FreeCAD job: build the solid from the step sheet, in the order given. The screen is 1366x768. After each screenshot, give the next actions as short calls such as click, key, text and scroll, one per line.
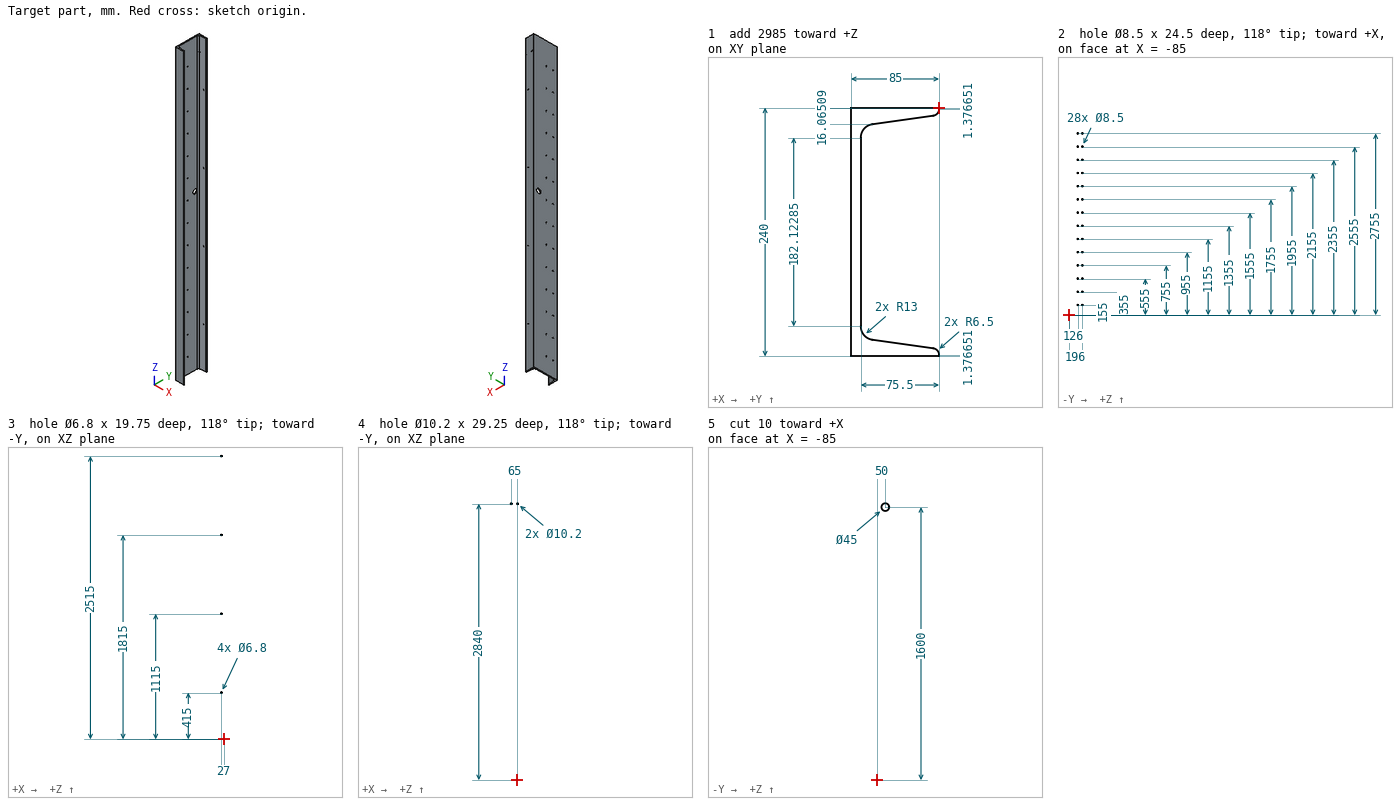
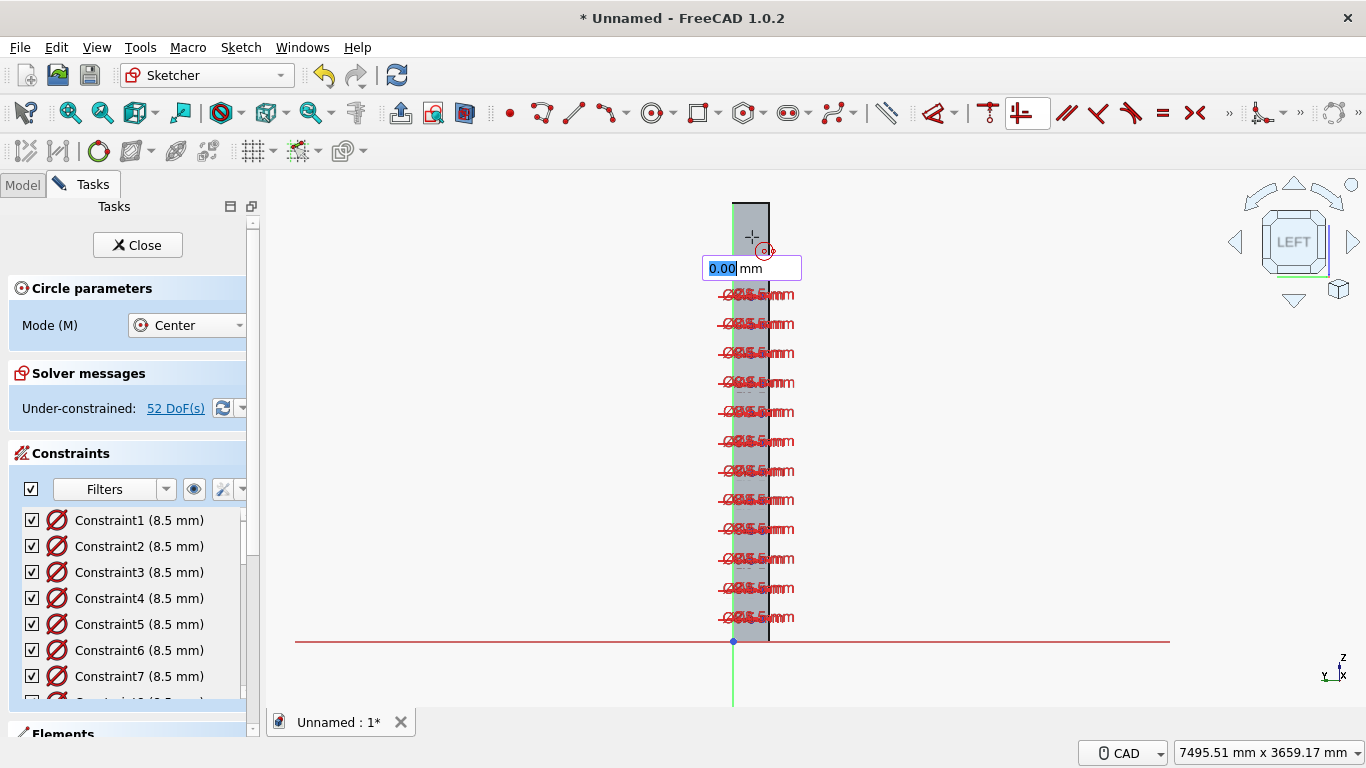
text(8.5)
key(Return)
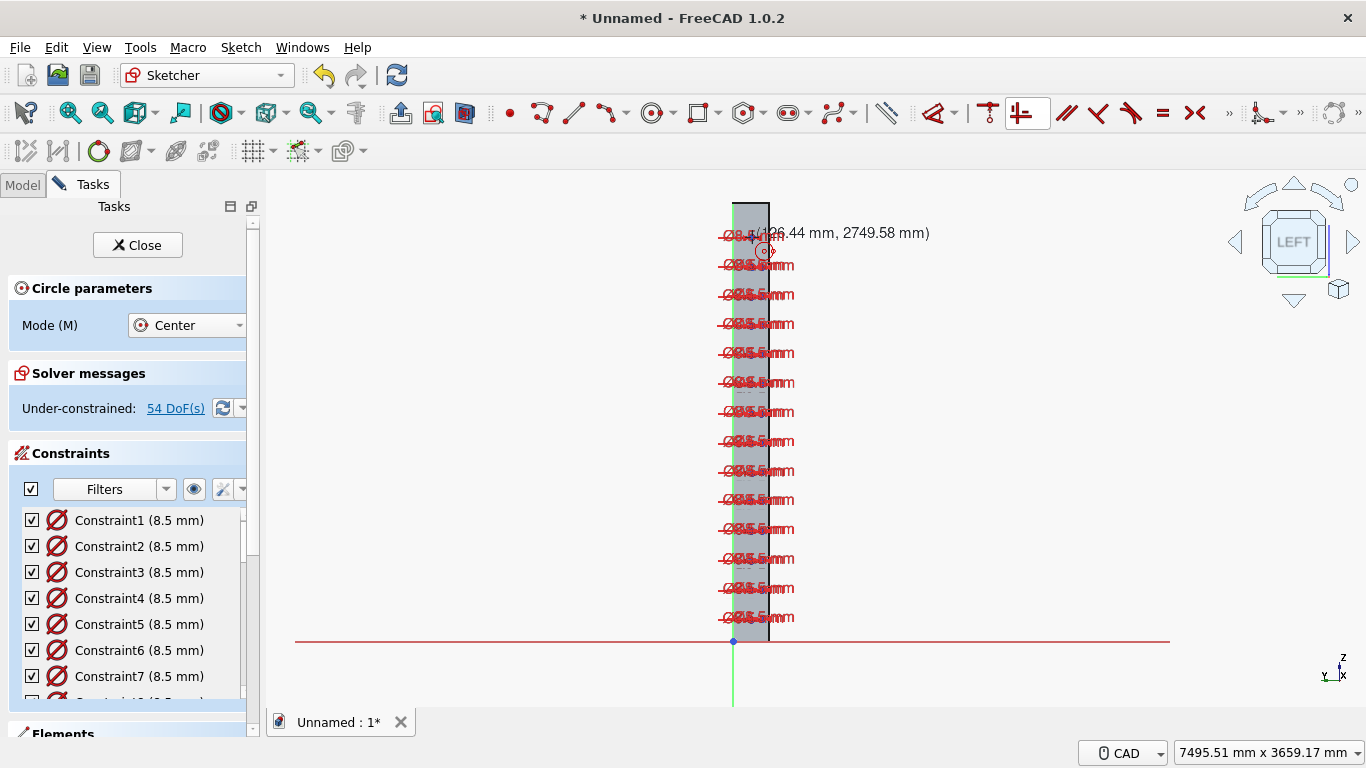
scroll(762, 237, up, 18)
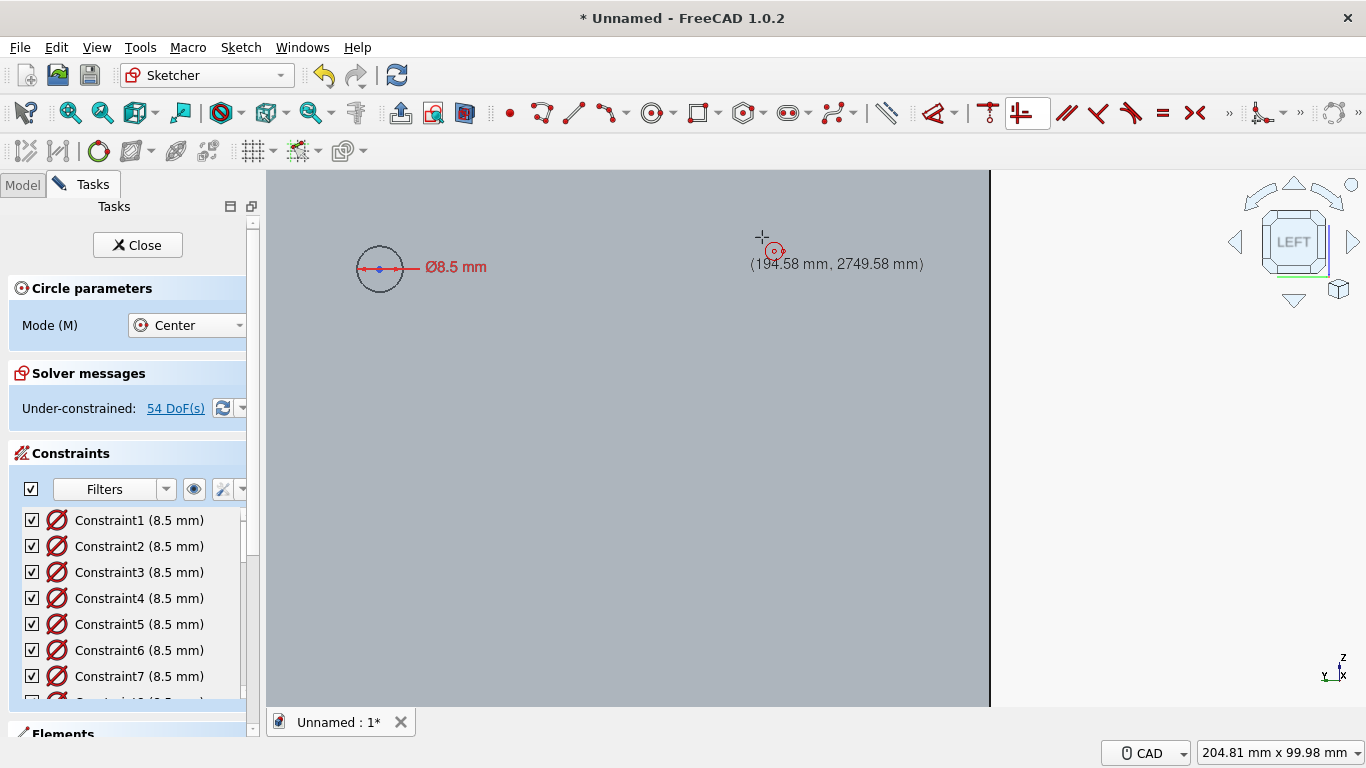
scroll(762, 237, down, 18)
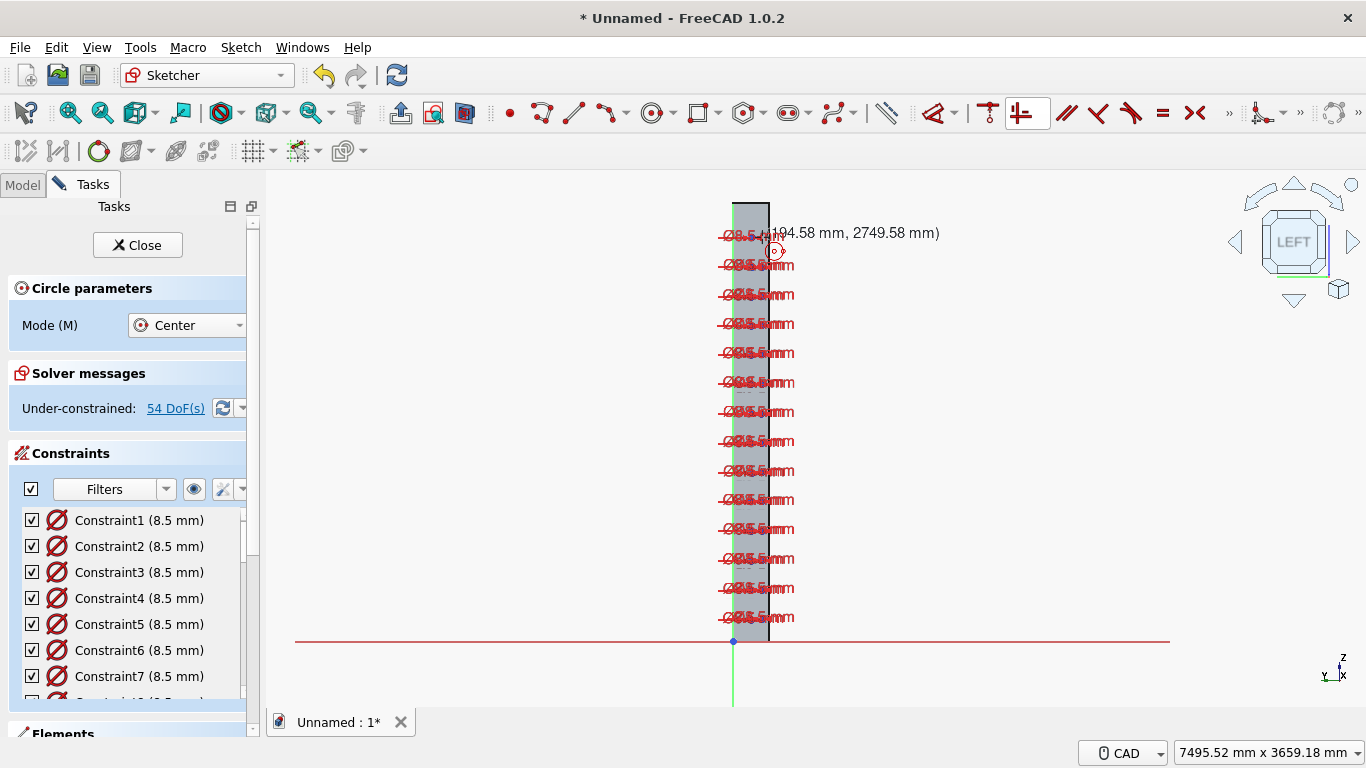
scroll(762, 237, up, 3)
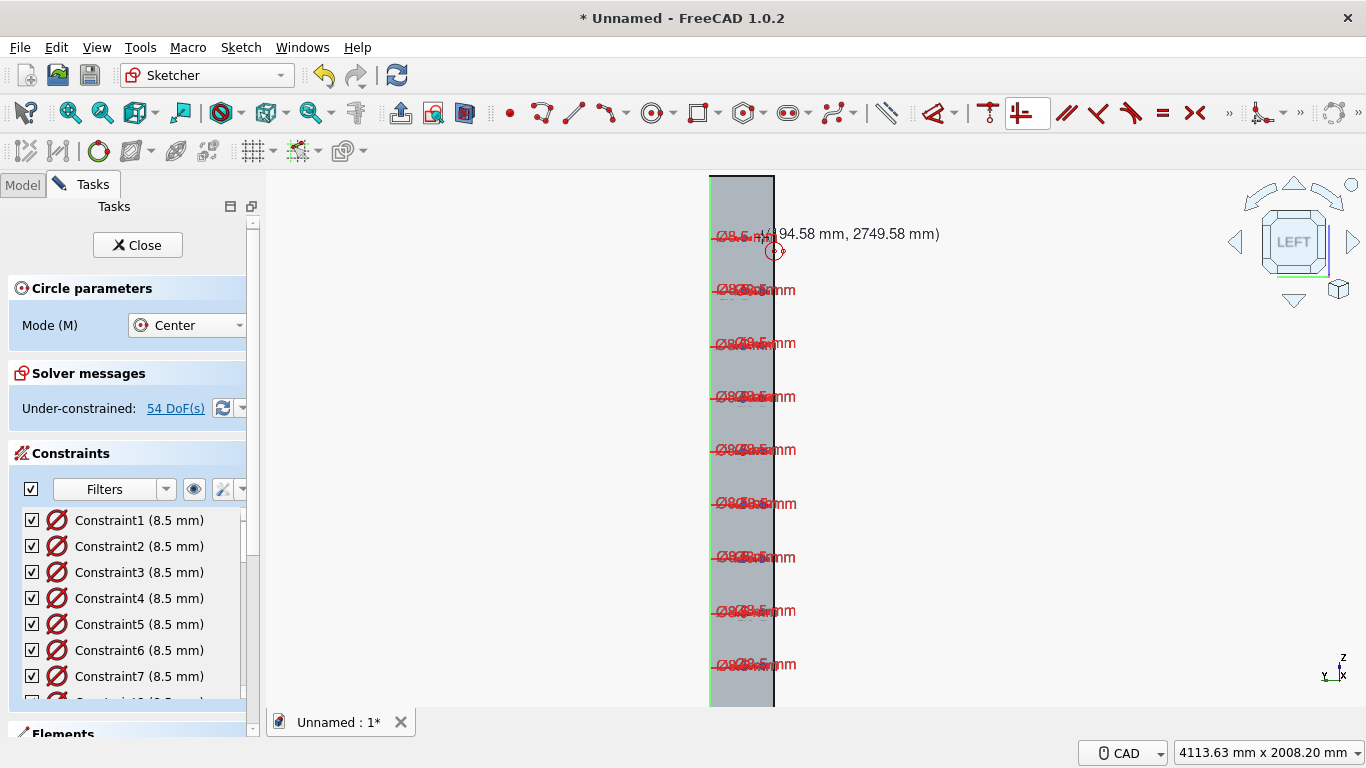
click(762, 237)
move(763, 236)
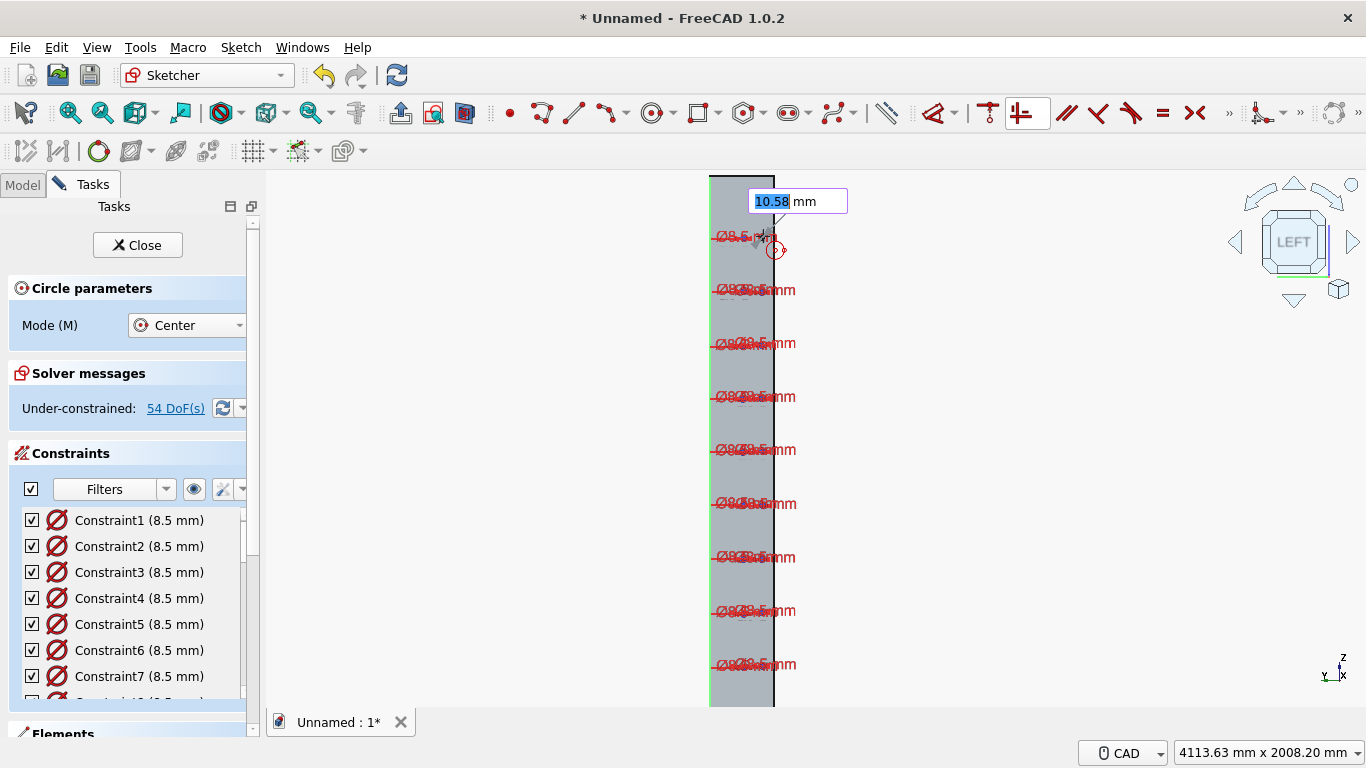
text(8.5)
key(Return)
key(Escape)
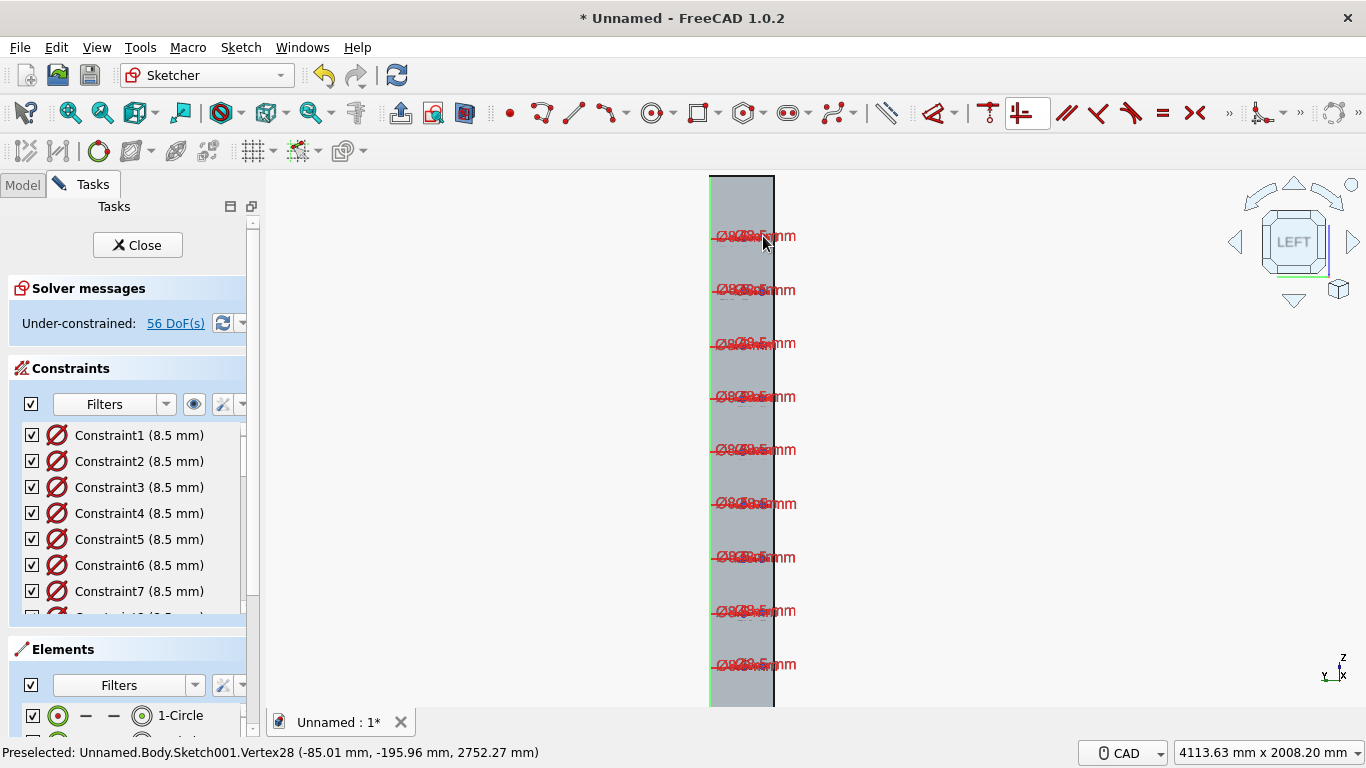
scroll(757, 303, down, 4)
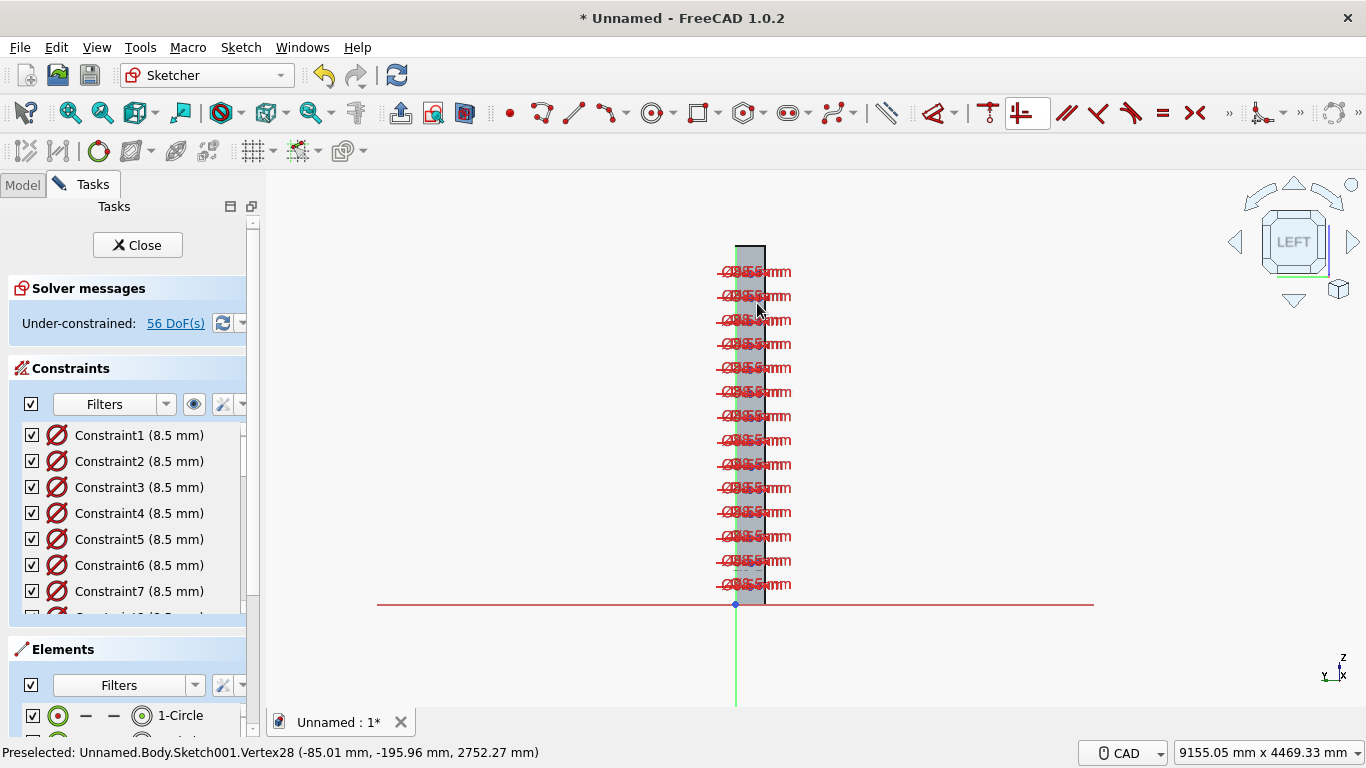
scroll(751, 587, up, 2)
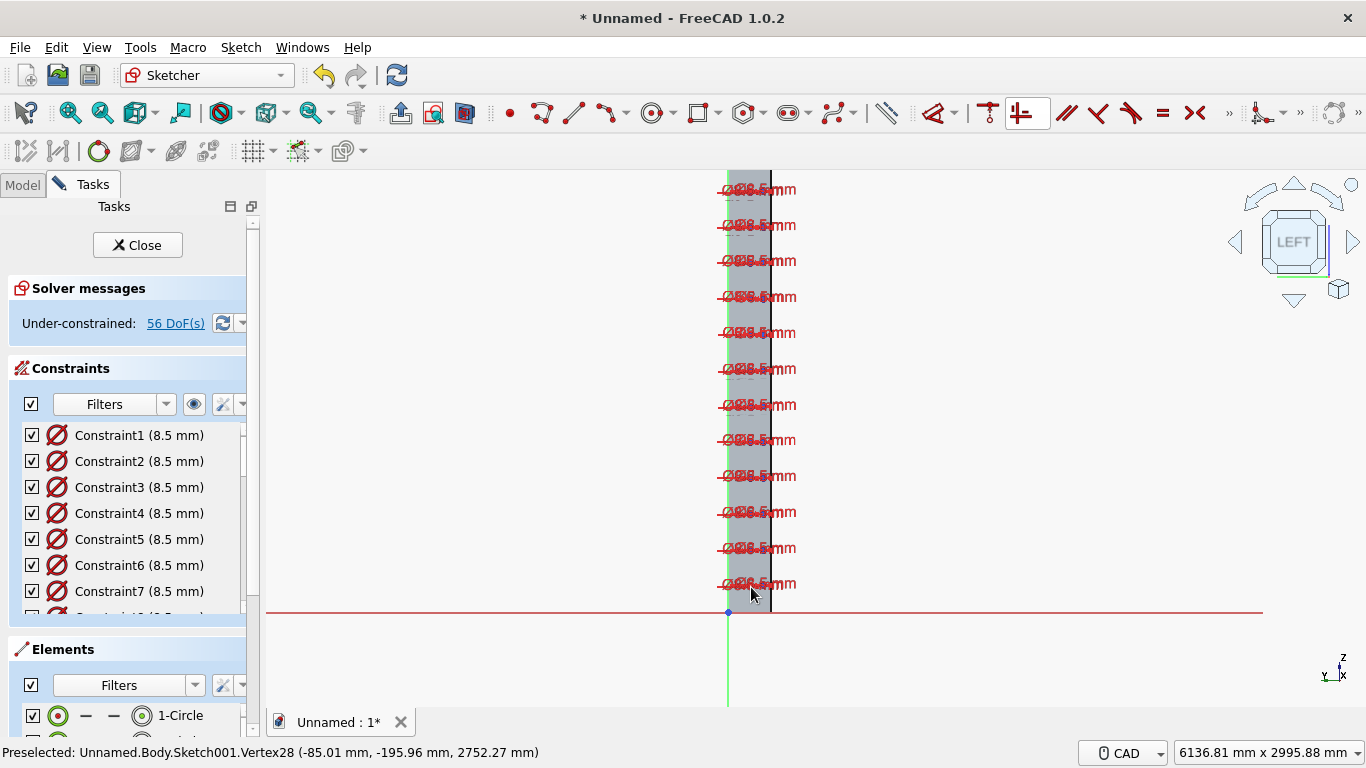
click(750, 587)